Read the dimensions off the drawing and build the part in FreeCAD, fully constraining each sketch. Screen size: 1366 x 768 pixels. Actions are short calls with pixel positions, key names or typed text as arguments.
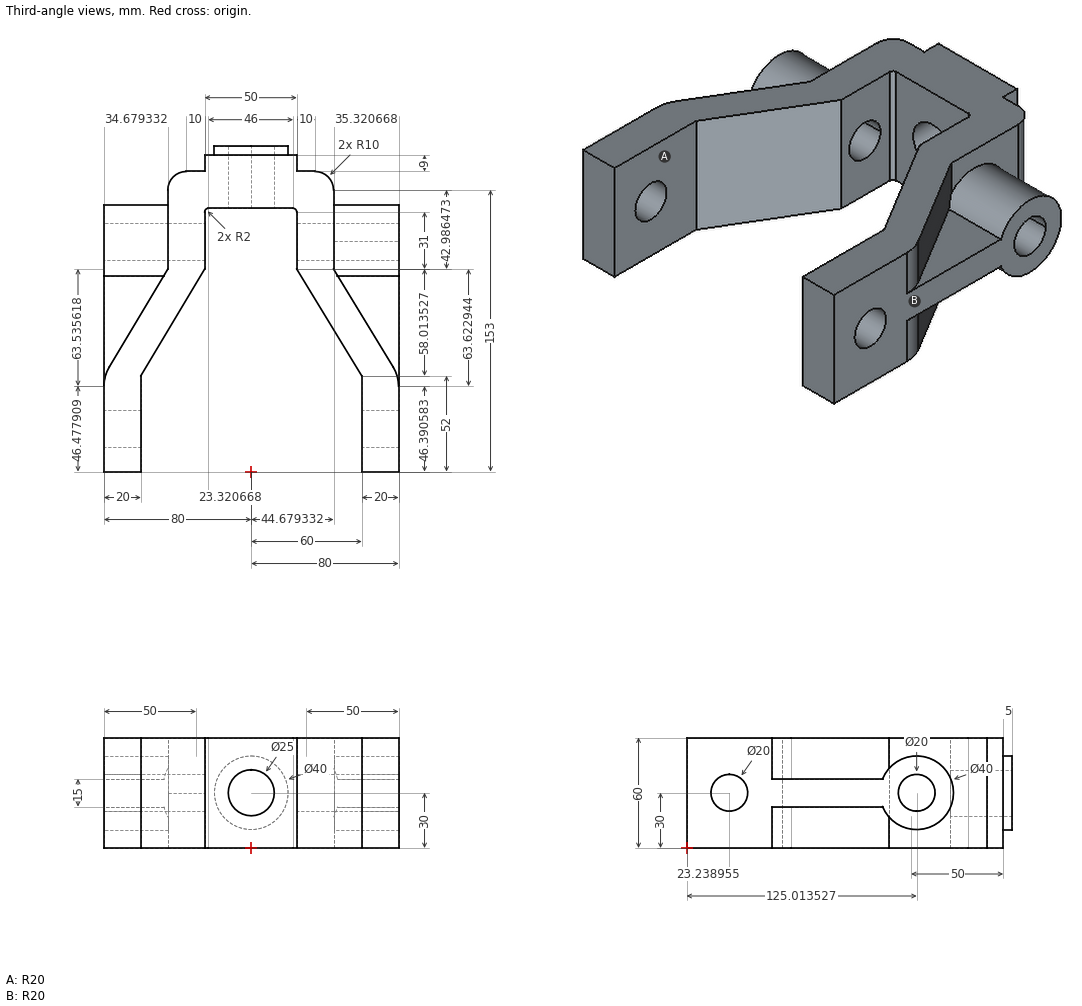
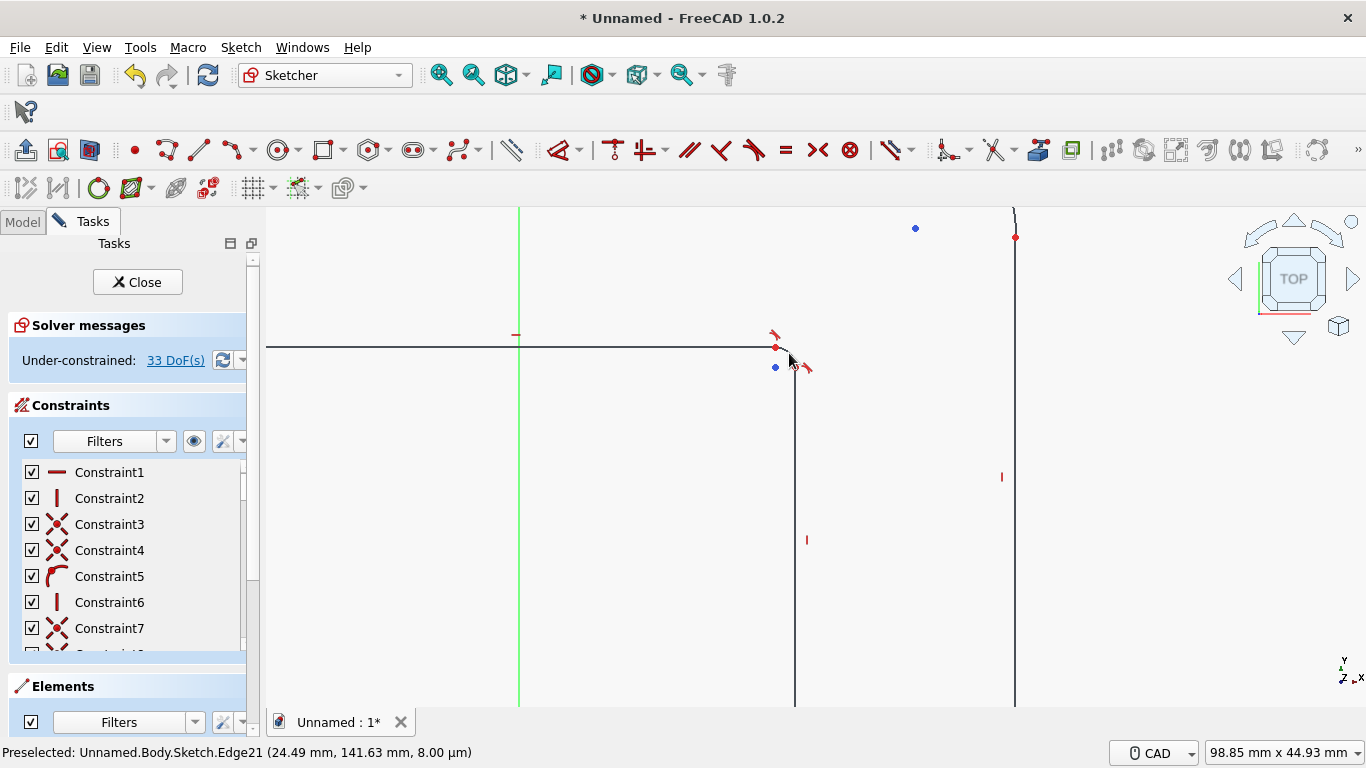
scroll(793, 354, down, 9)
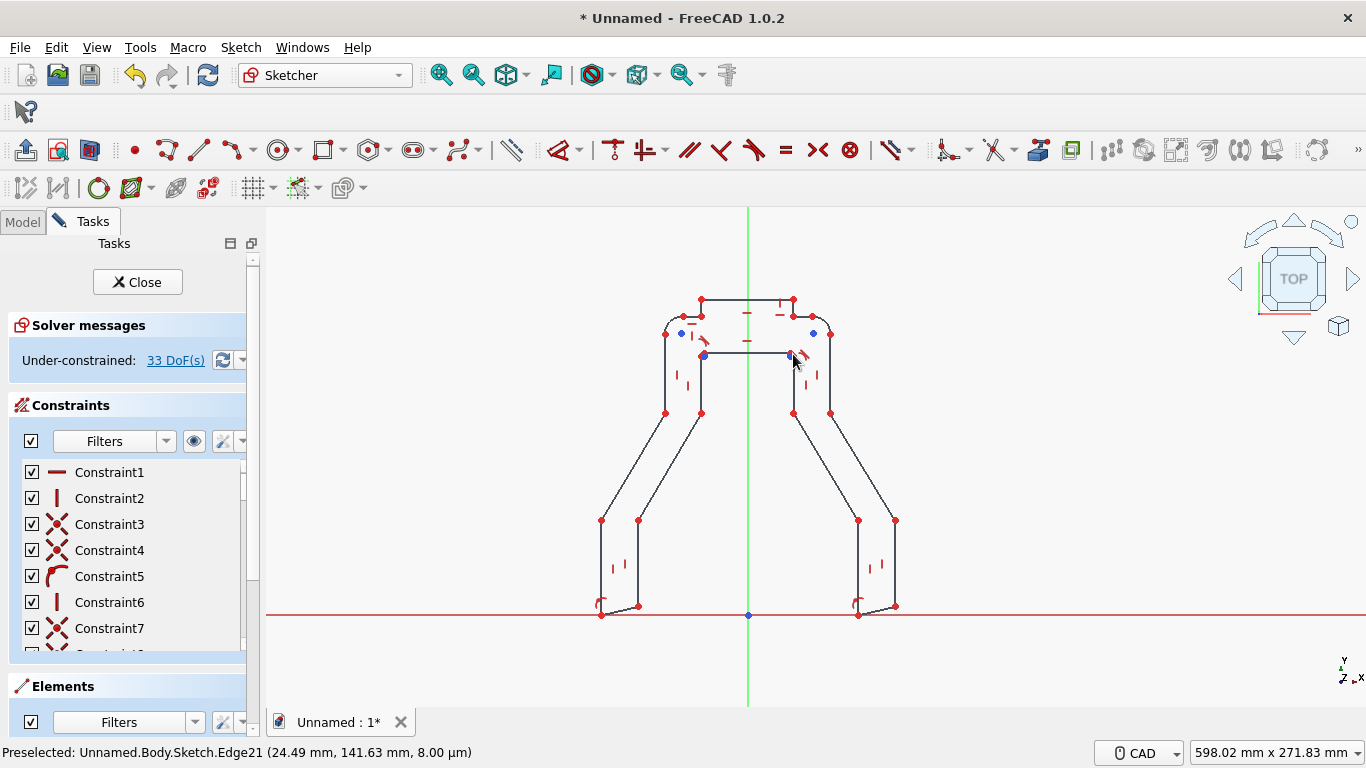
click(830, 390)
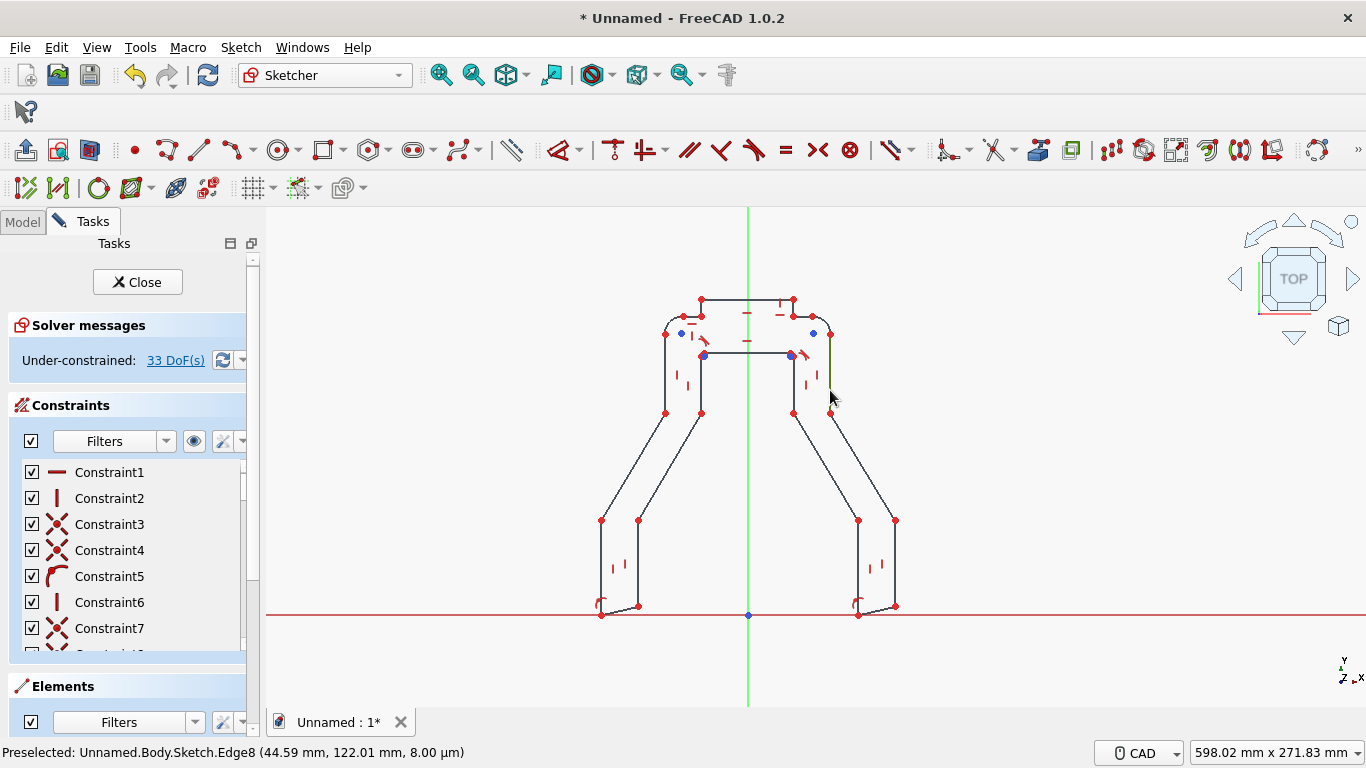
click(825, 322)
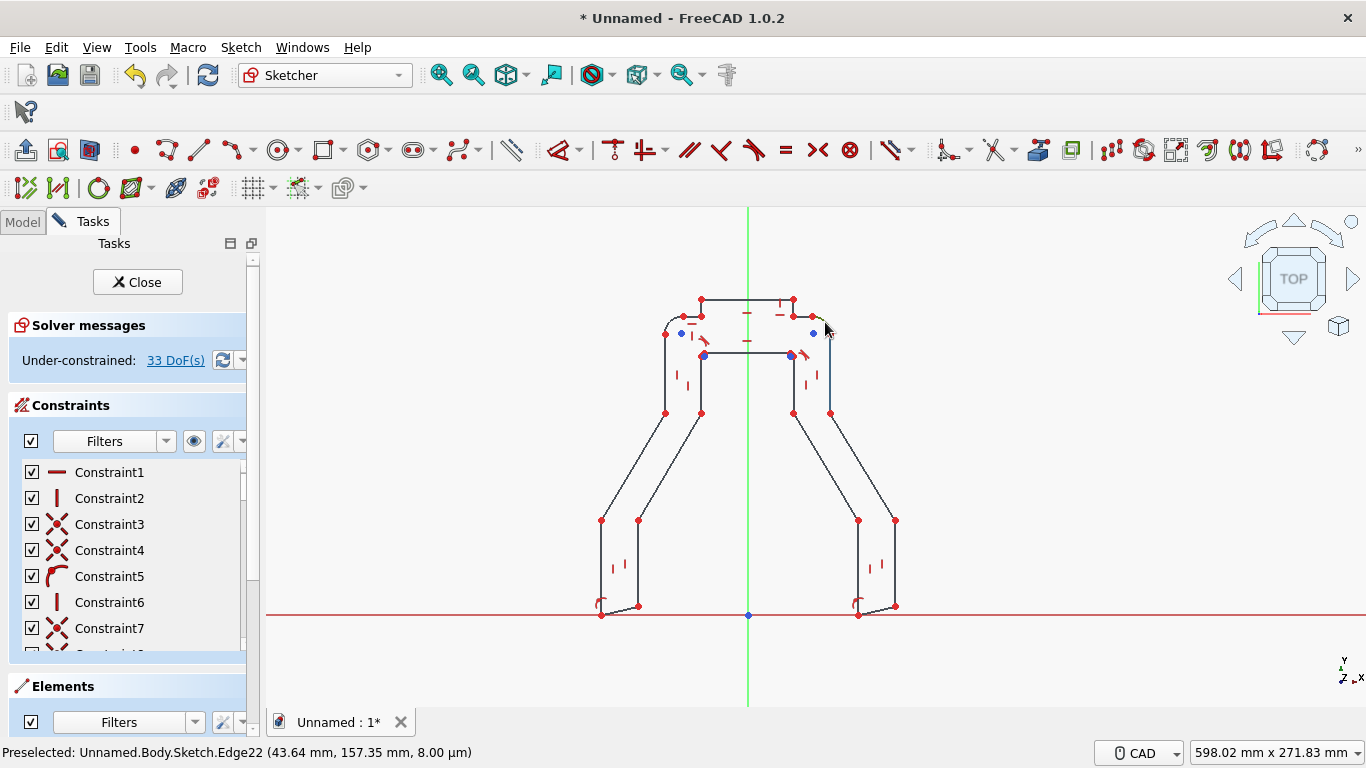
click(754, 150)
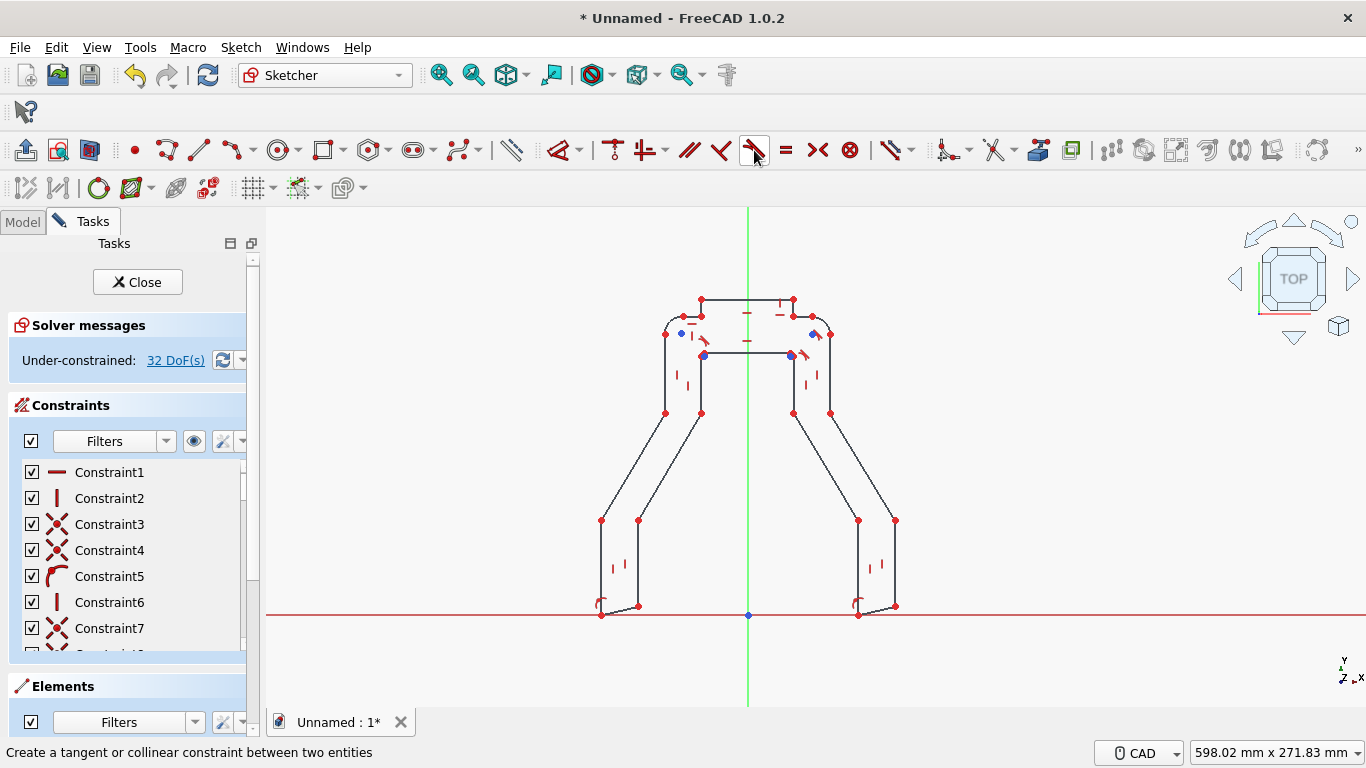
scroll(803, 317, up, 2)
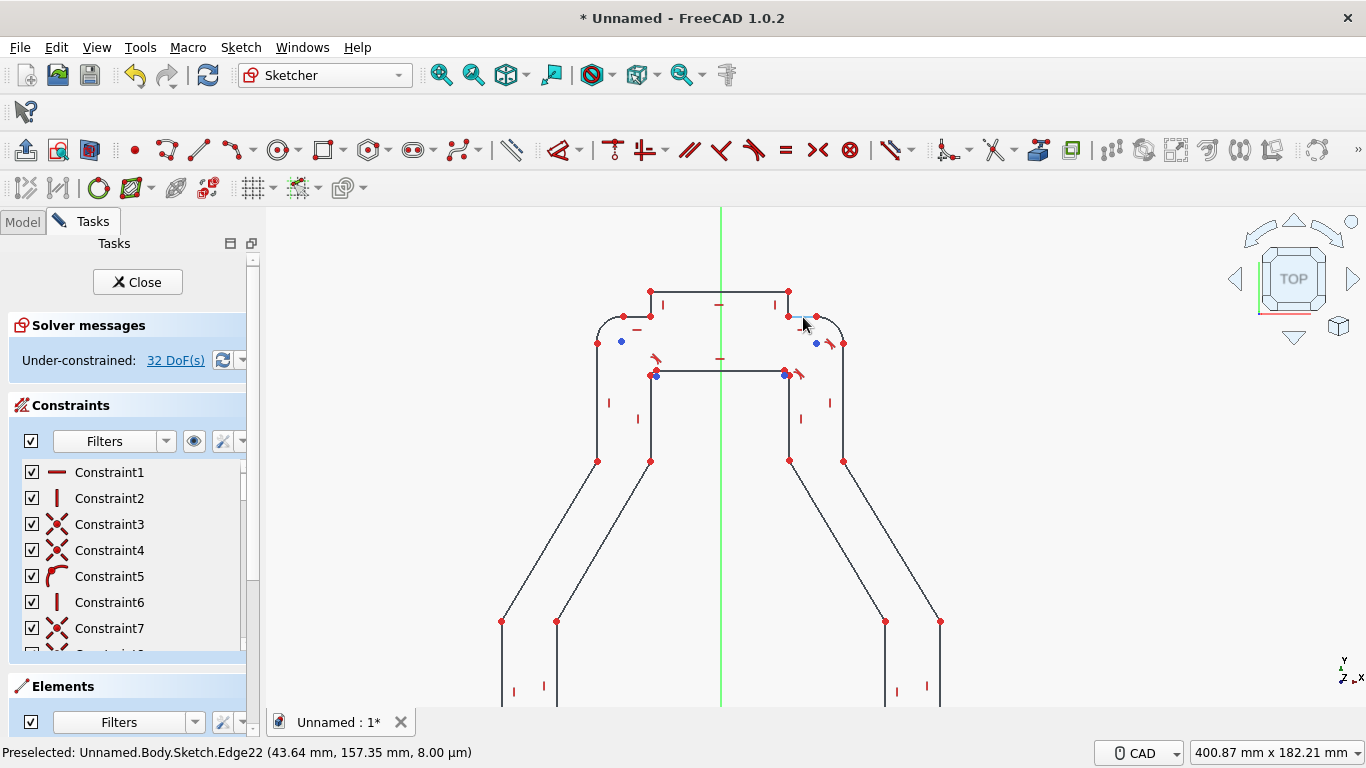
click(802, 317)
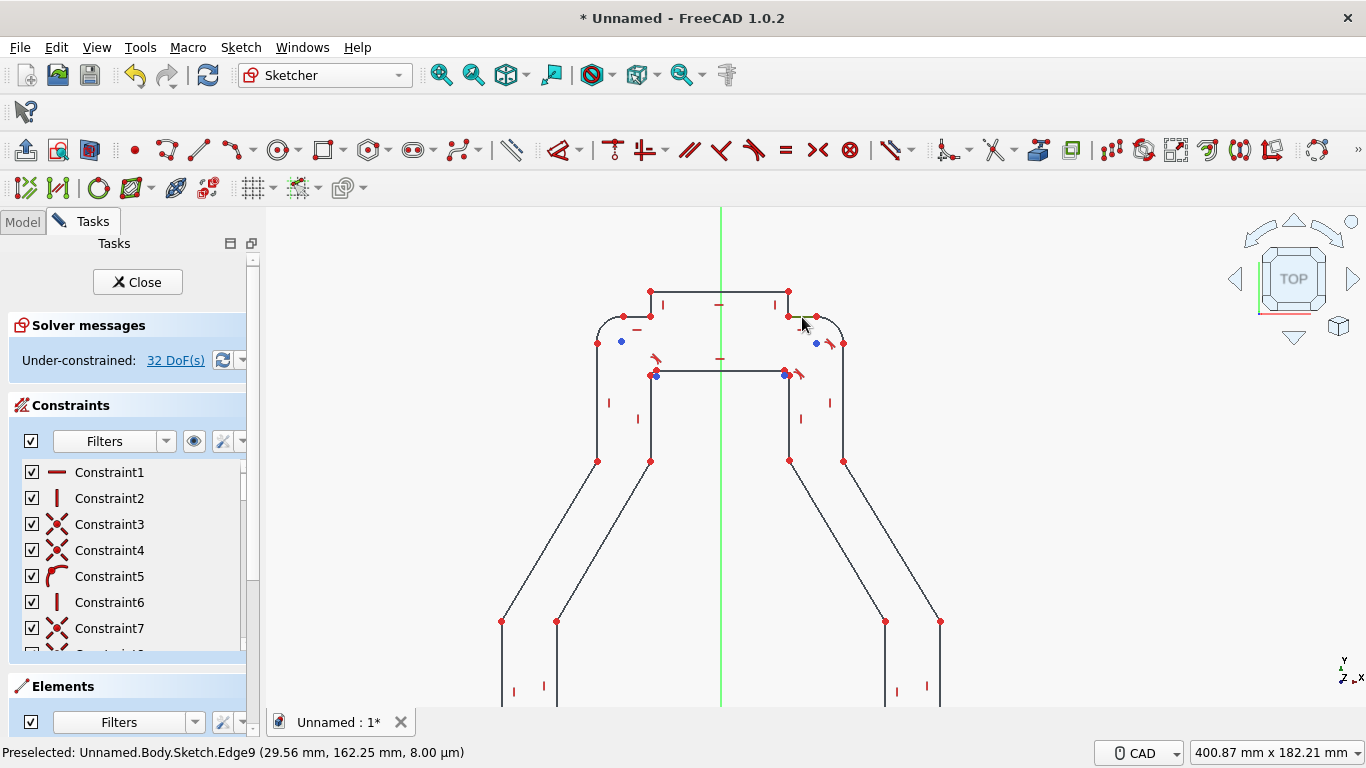
click(840, 332)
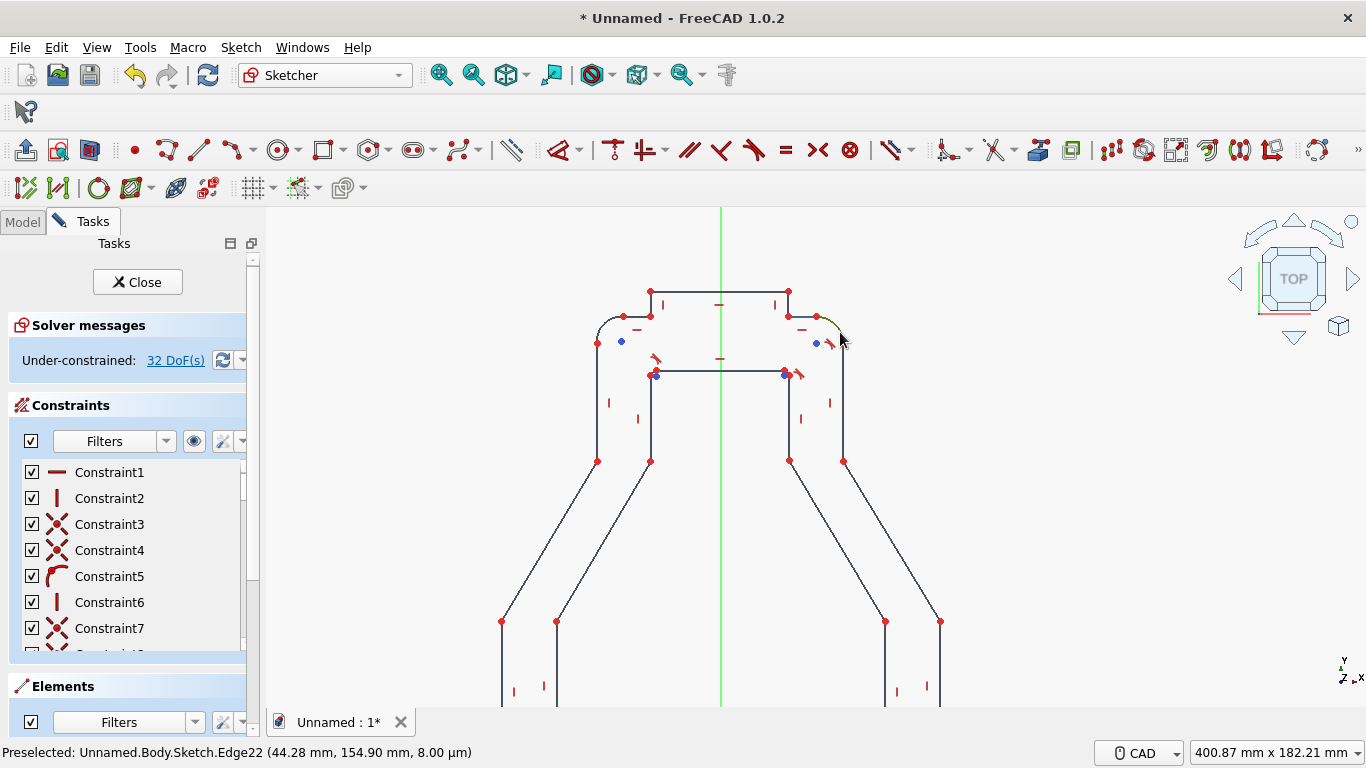
key(t)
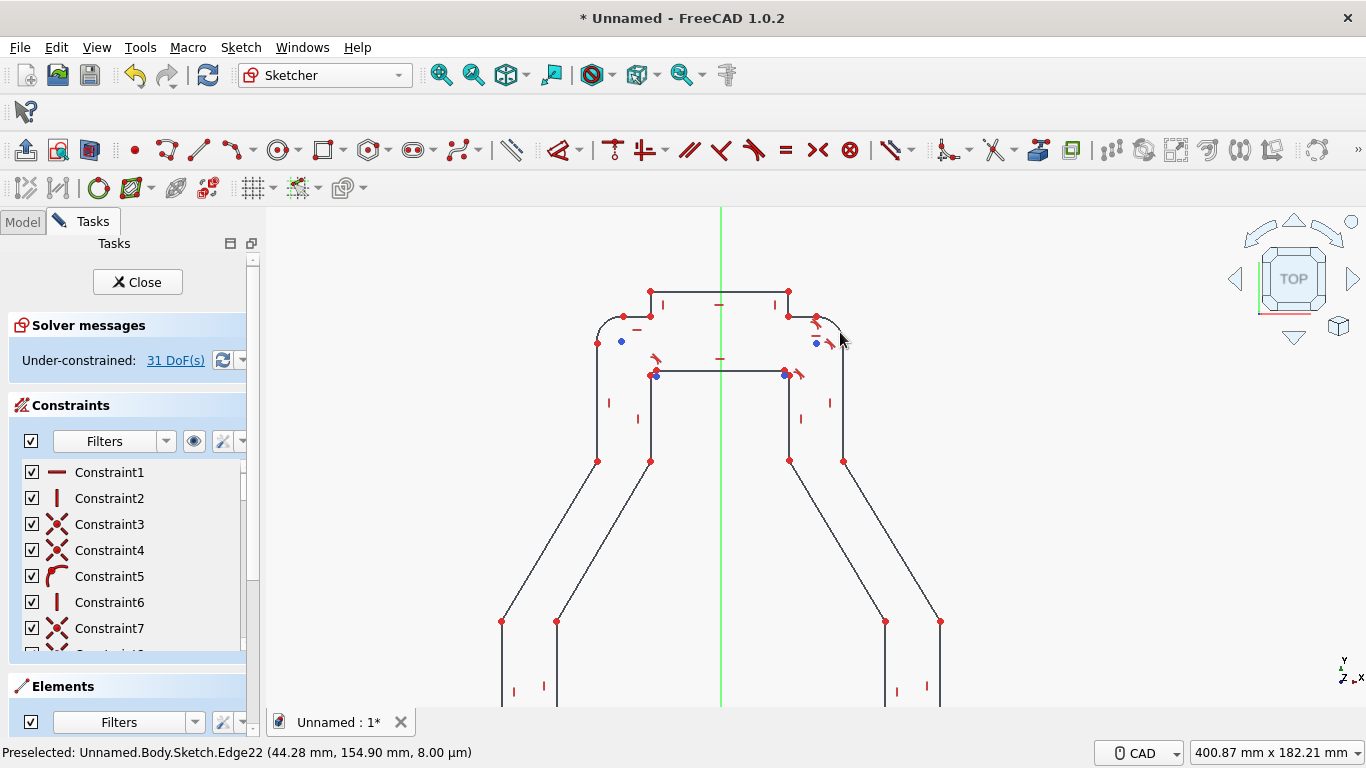
scroll(640, 317, up, 2)